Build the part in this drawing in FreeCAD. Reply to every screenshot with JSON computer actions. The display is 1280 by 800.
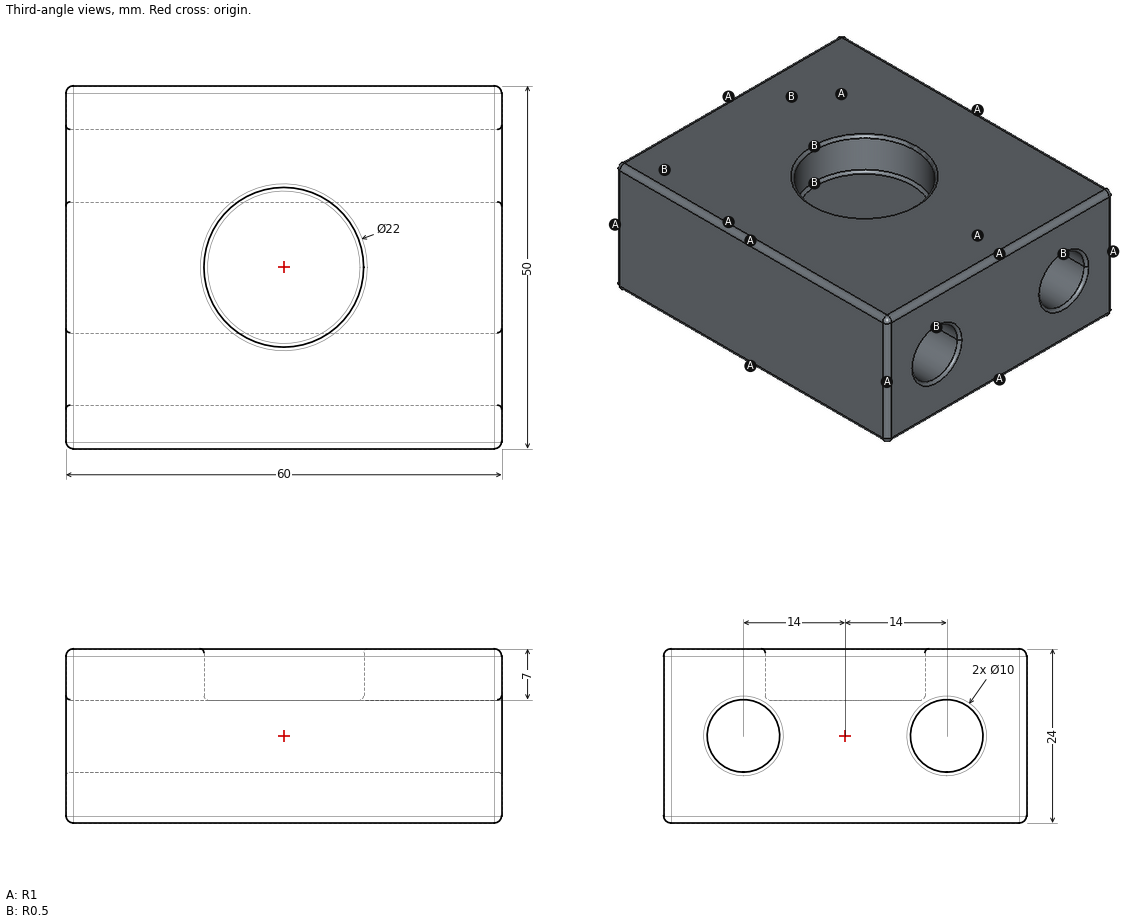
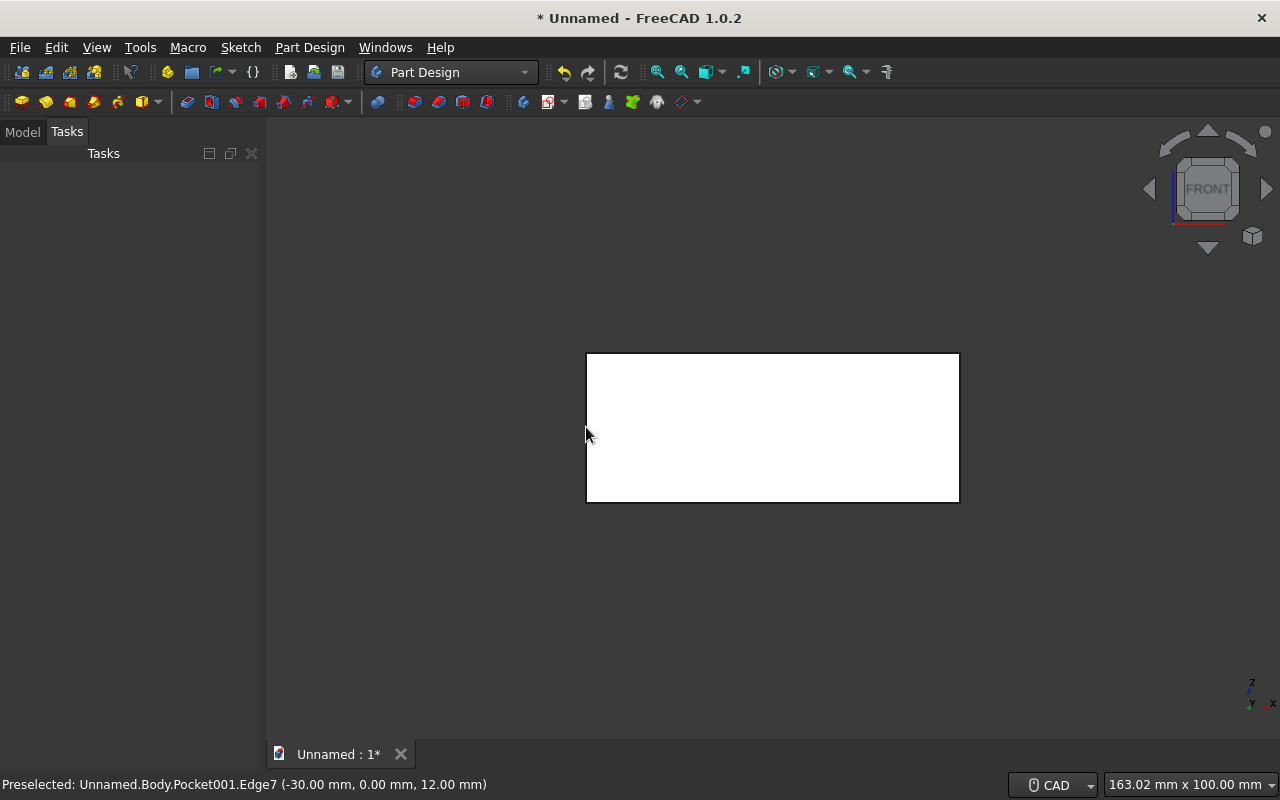
{"action": "left_click", "coordinate": [658, 72]}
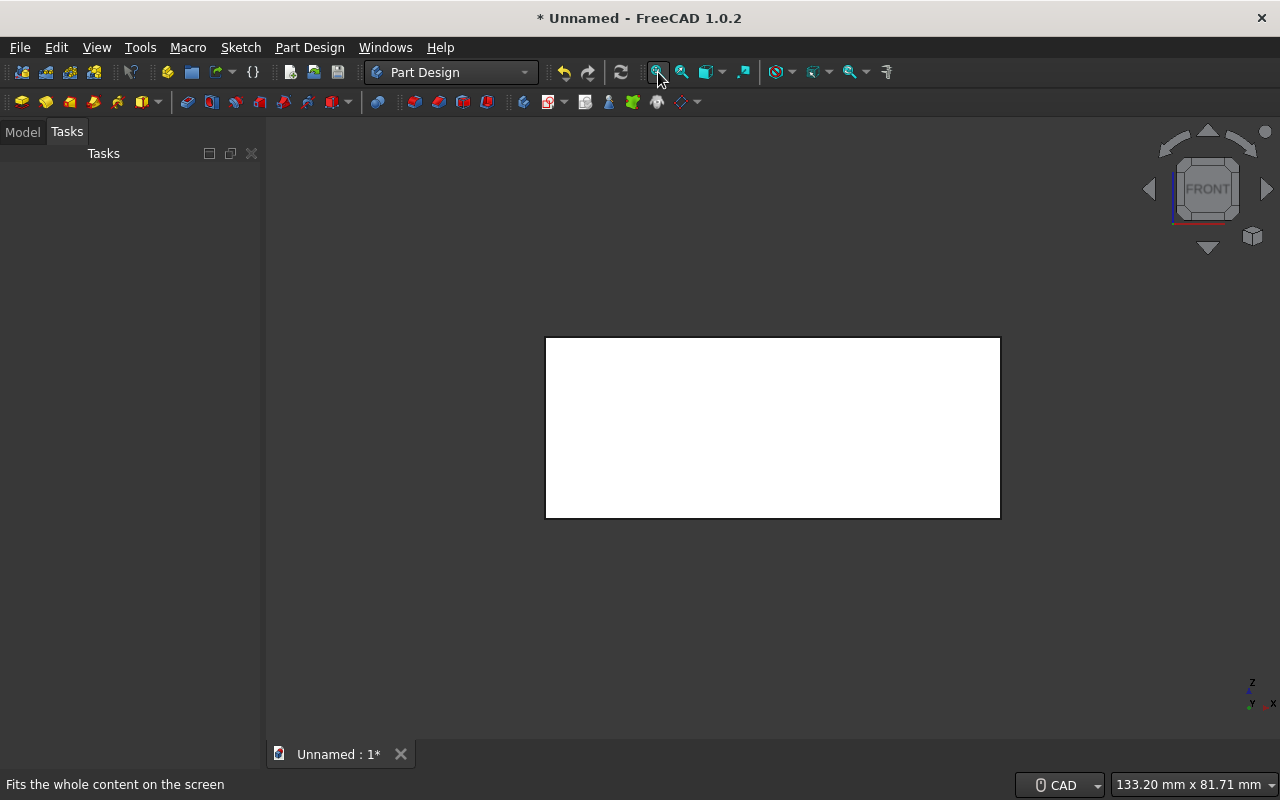
{"action": "key", "text": "3"}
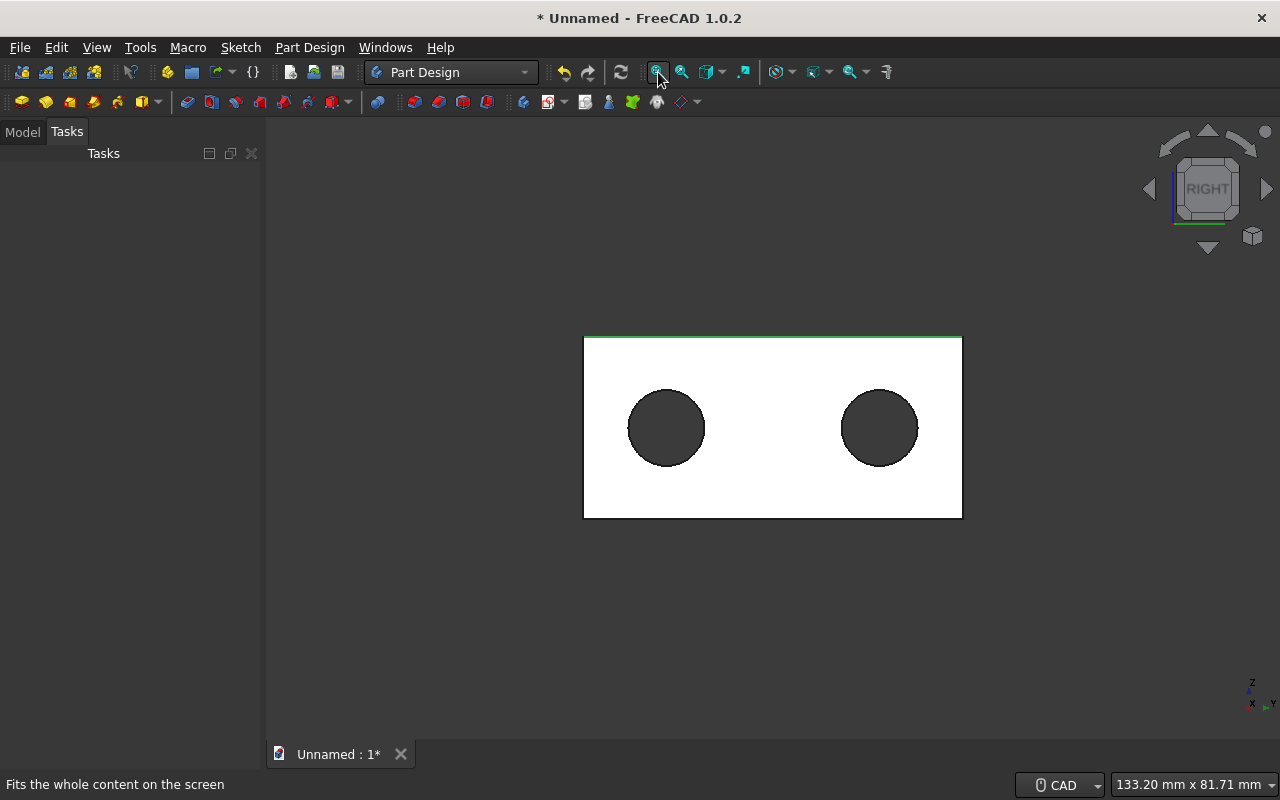
{"action": "left_click", "coordinate": [658, 72]}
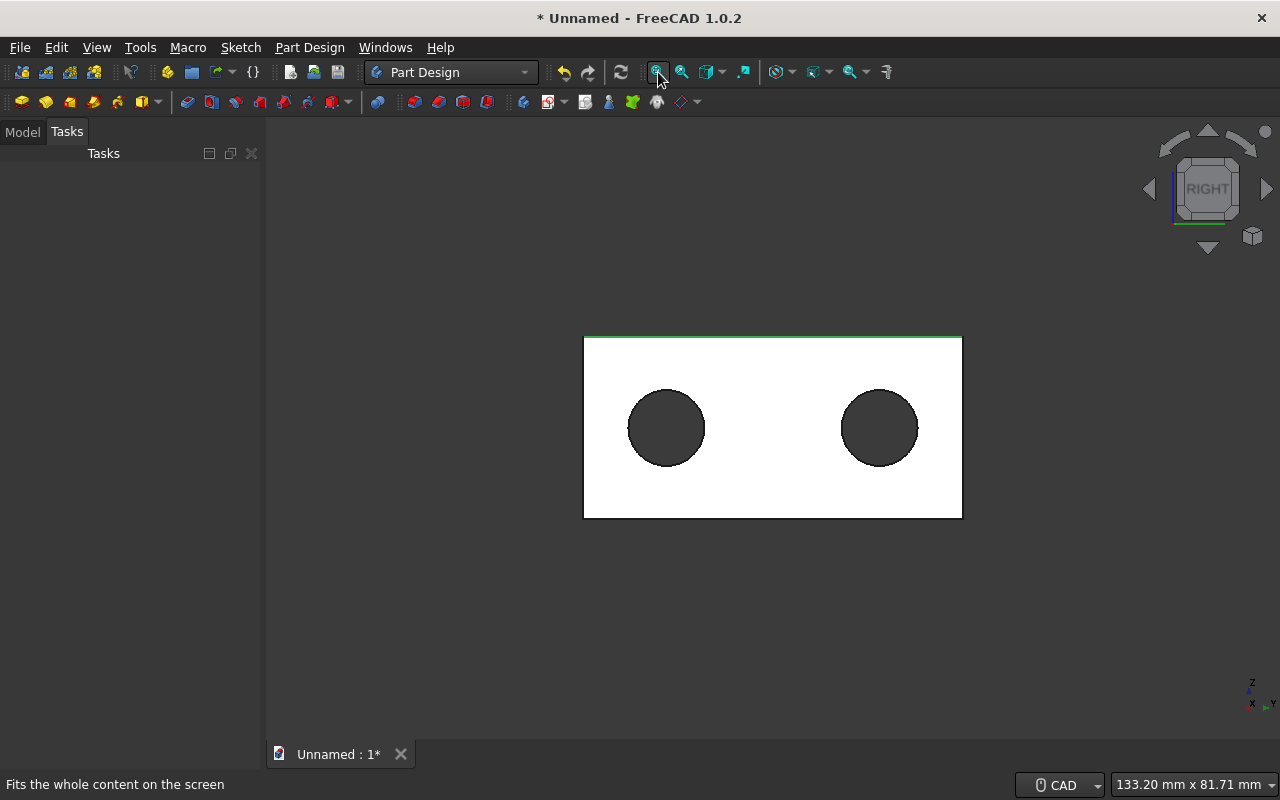
{"action": "key", "text": "5"}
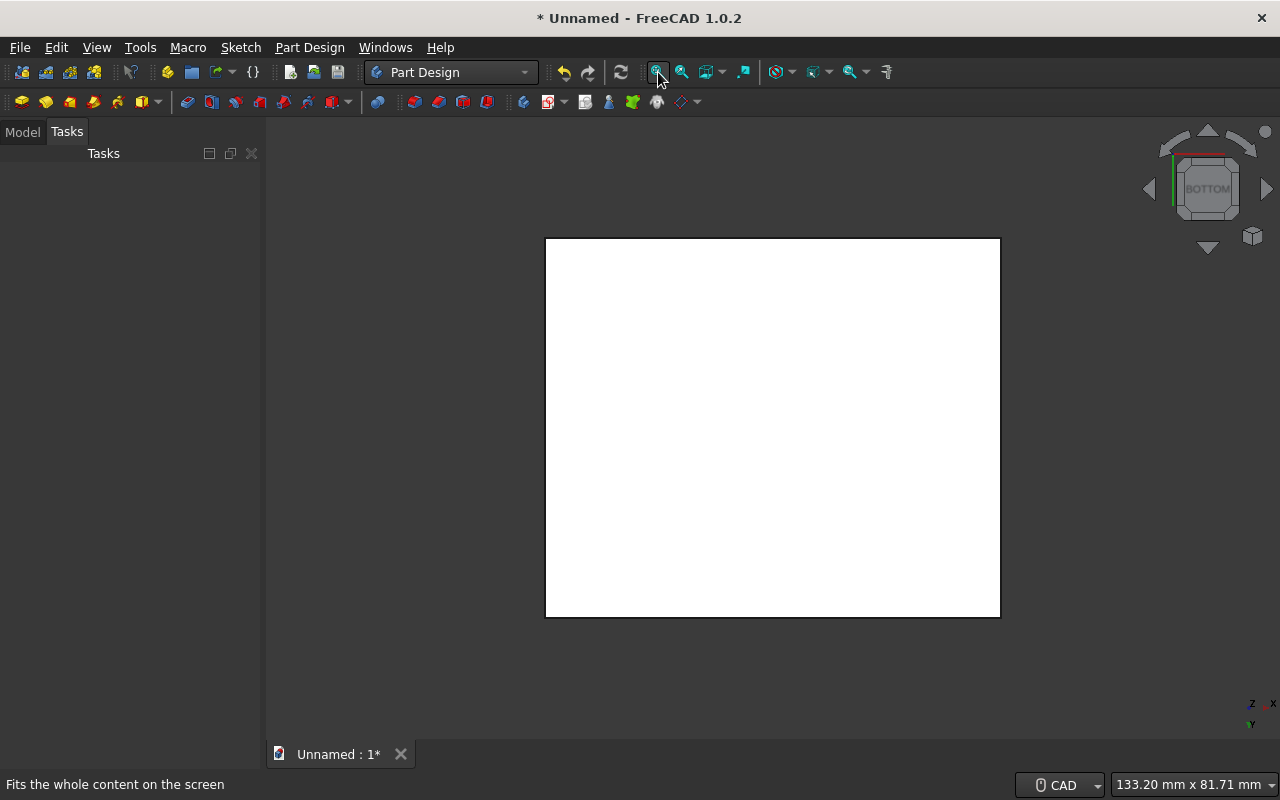
{"action": "left_click", "coordinate": [773, 427], "text": "ctrl"}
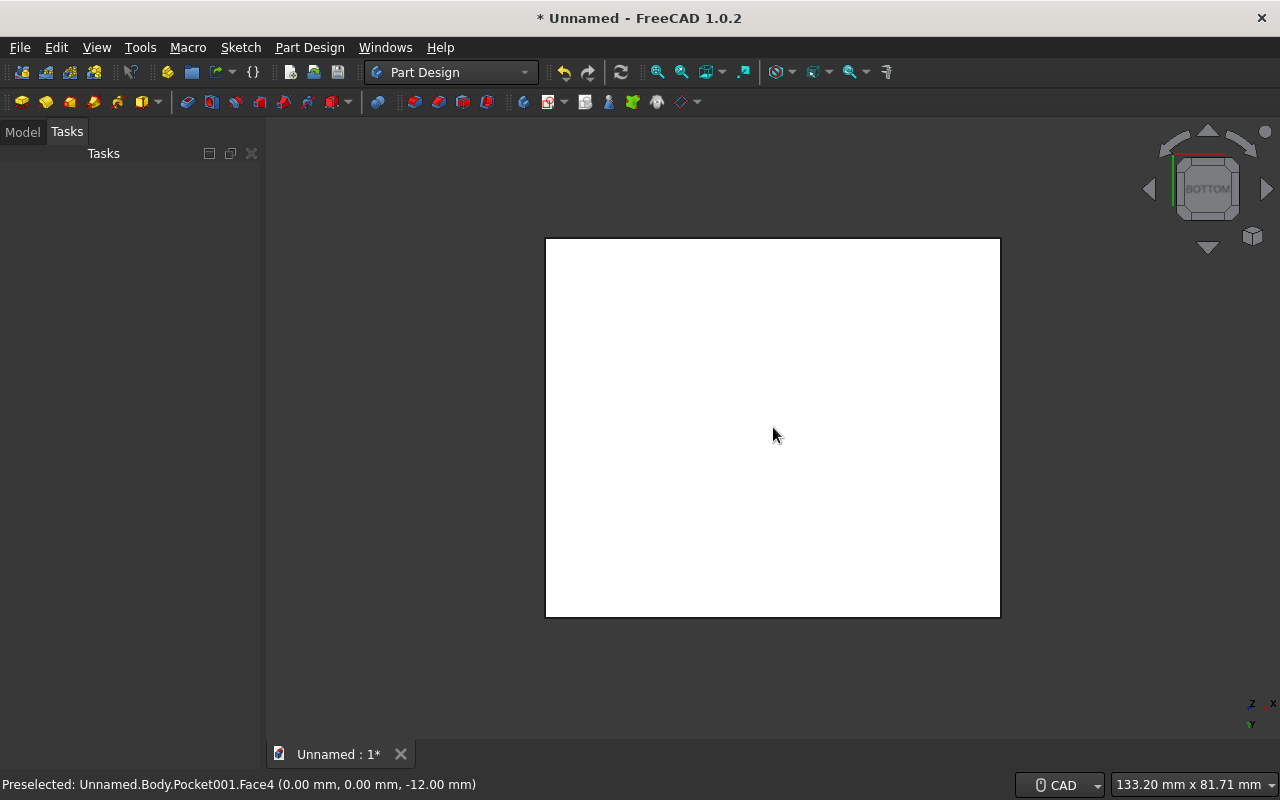
{"action": "key", "text": "4"}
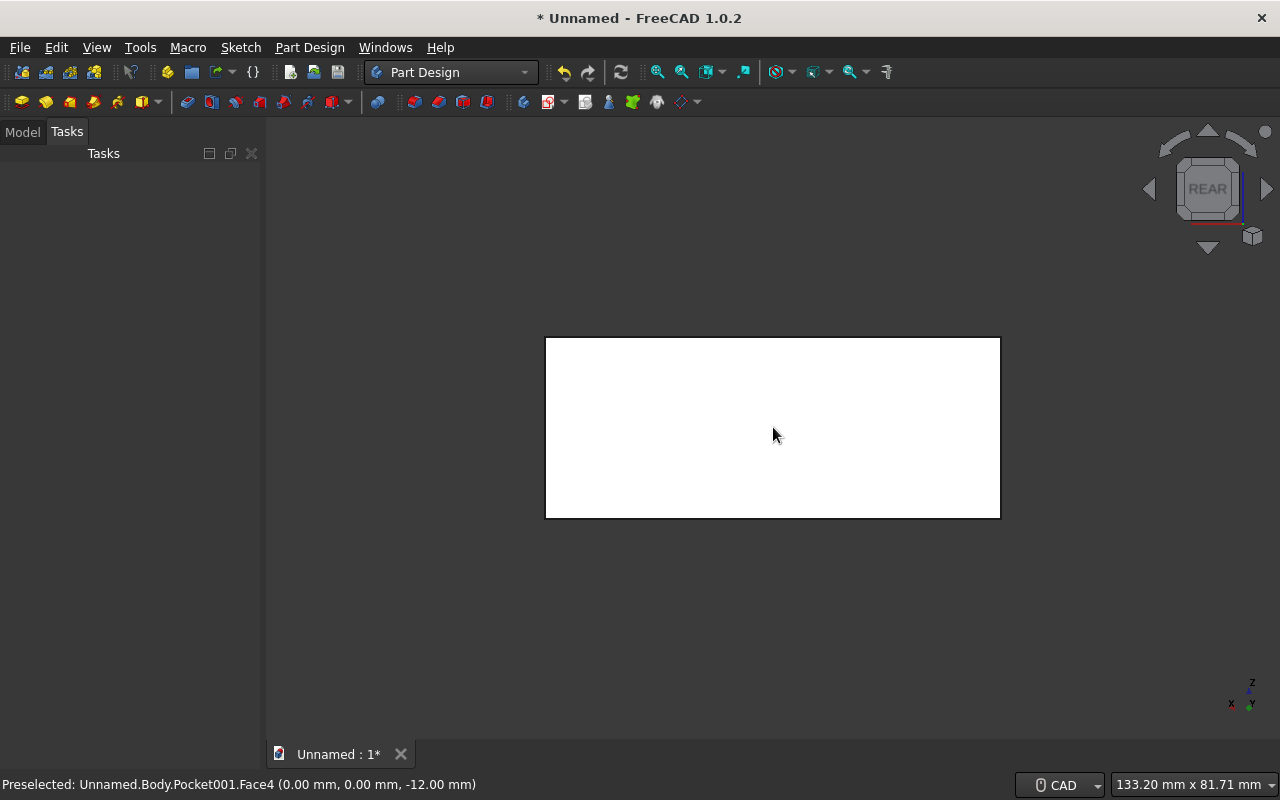
{"action": "left_click", "coordinate": [658, 72]}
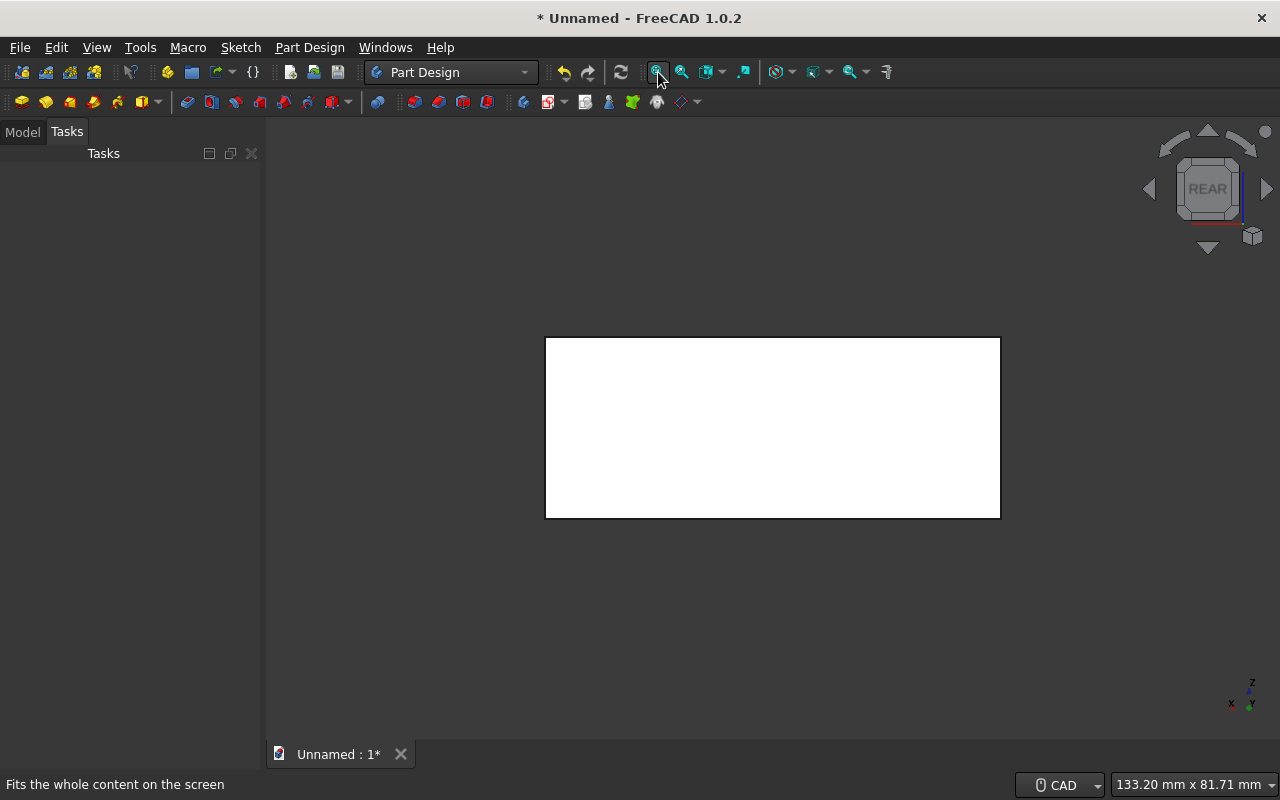
{"action": "left_click", "coordinate": [642, 427], "text": "ctrl"}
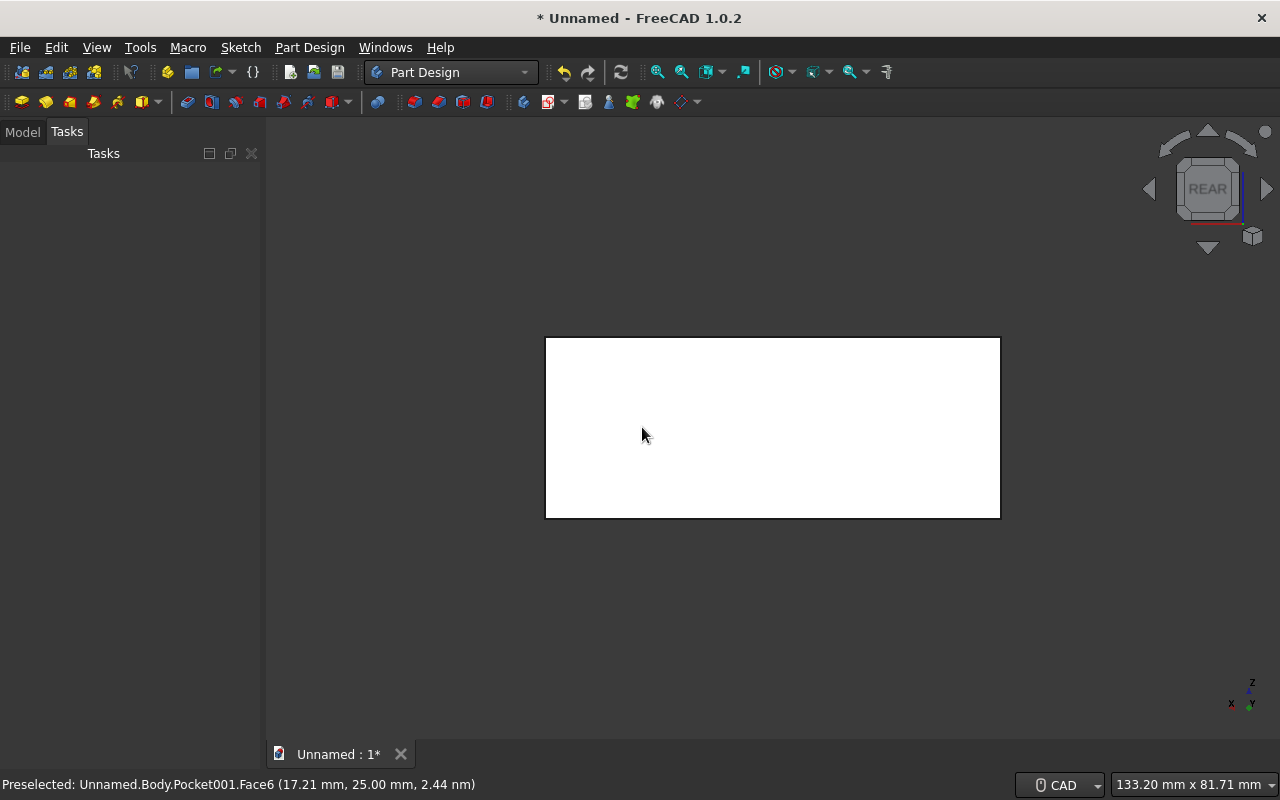
{"action": "left_click", "coordinate": [416, 102]}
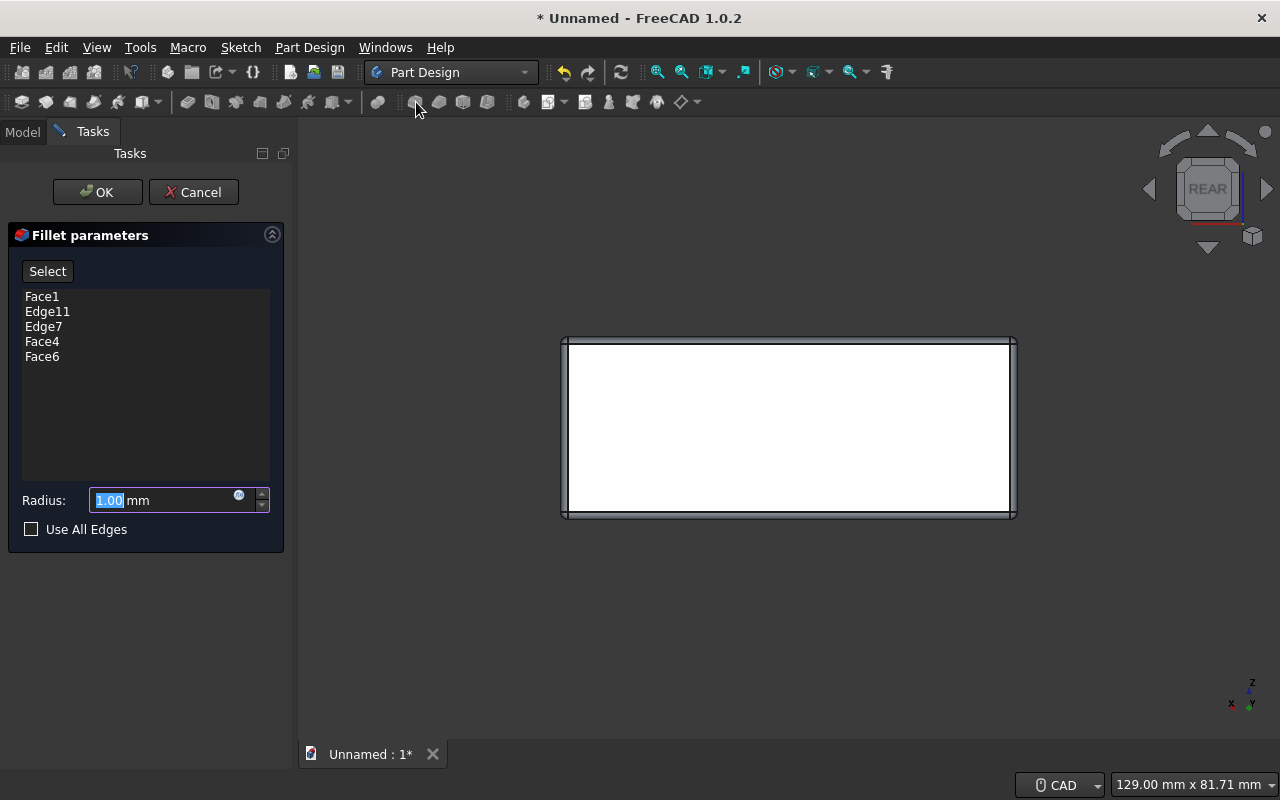
{"action": "type", "text": "1"}
{"action": "key", "text": "Tab"}